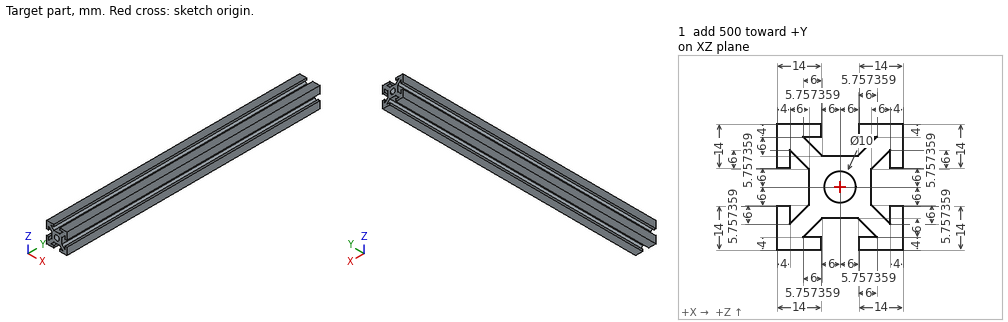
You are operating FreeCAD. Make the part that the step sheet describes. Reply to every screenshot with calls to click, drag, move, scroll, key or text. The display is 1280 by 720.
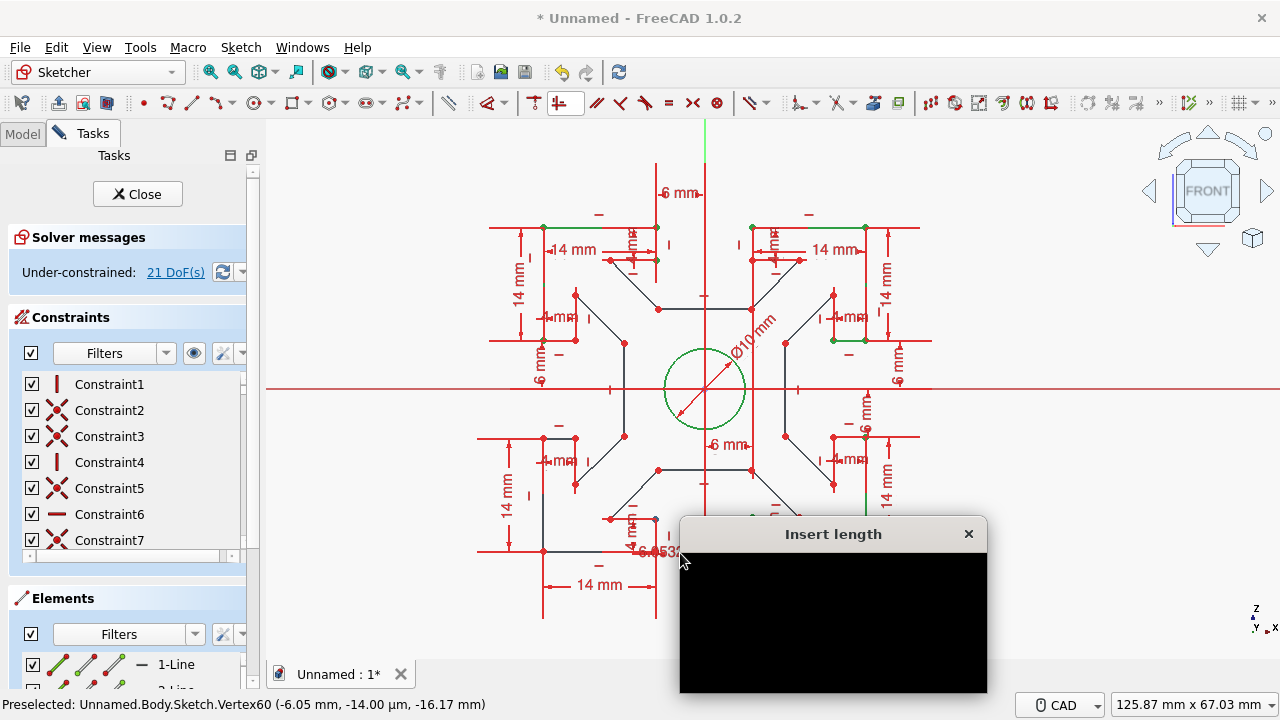
text(6)
key(Return)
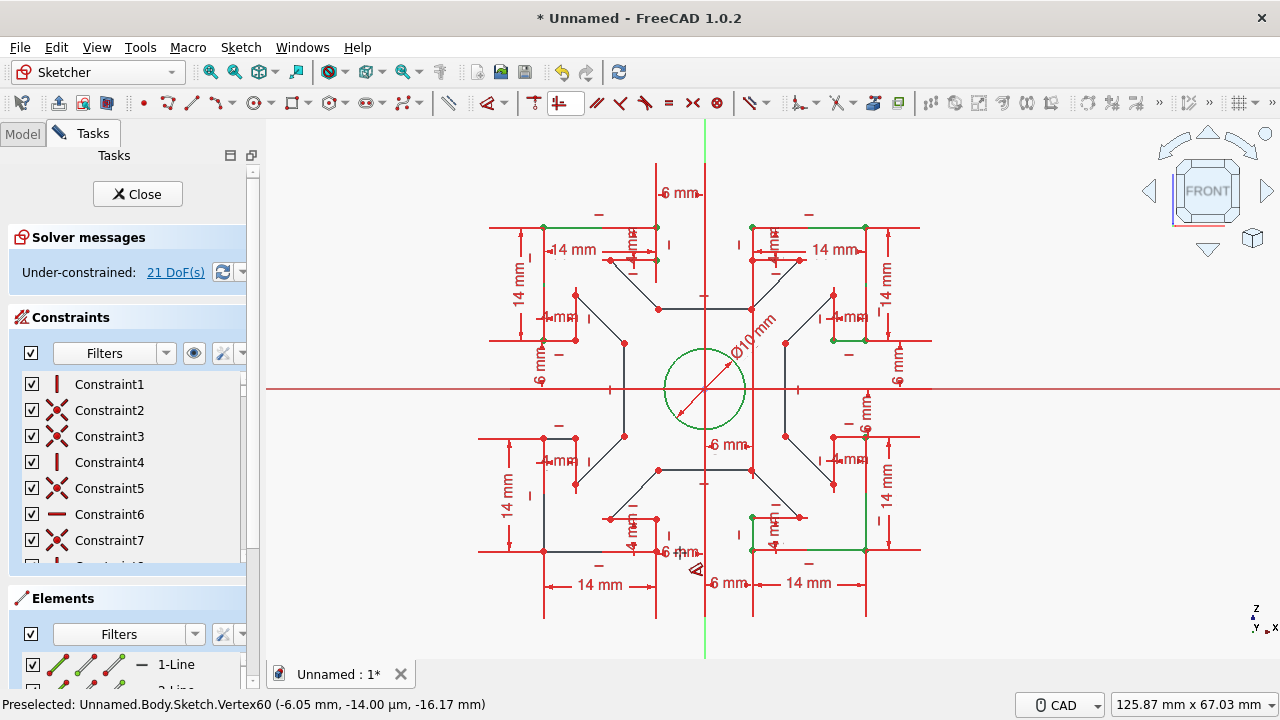
click(544, 439)
click(510, 414)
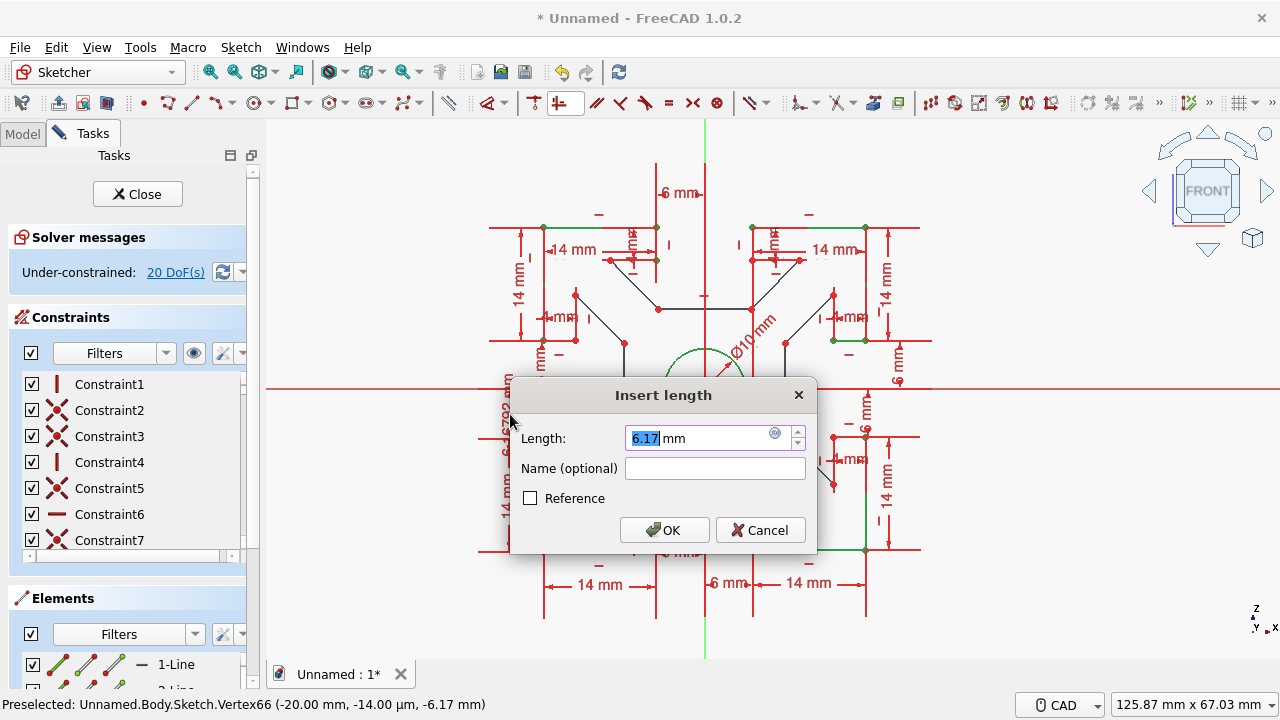
text(6)
key(Return)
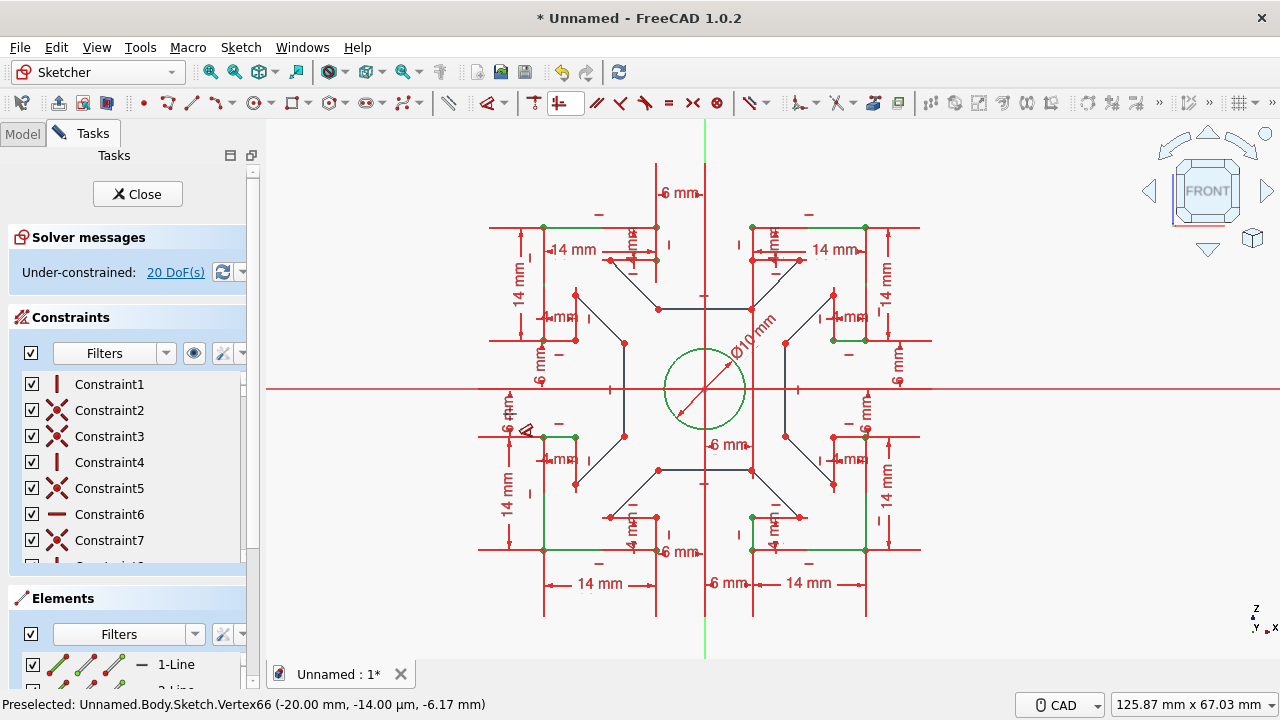
click(610, 329)
click(600, 213)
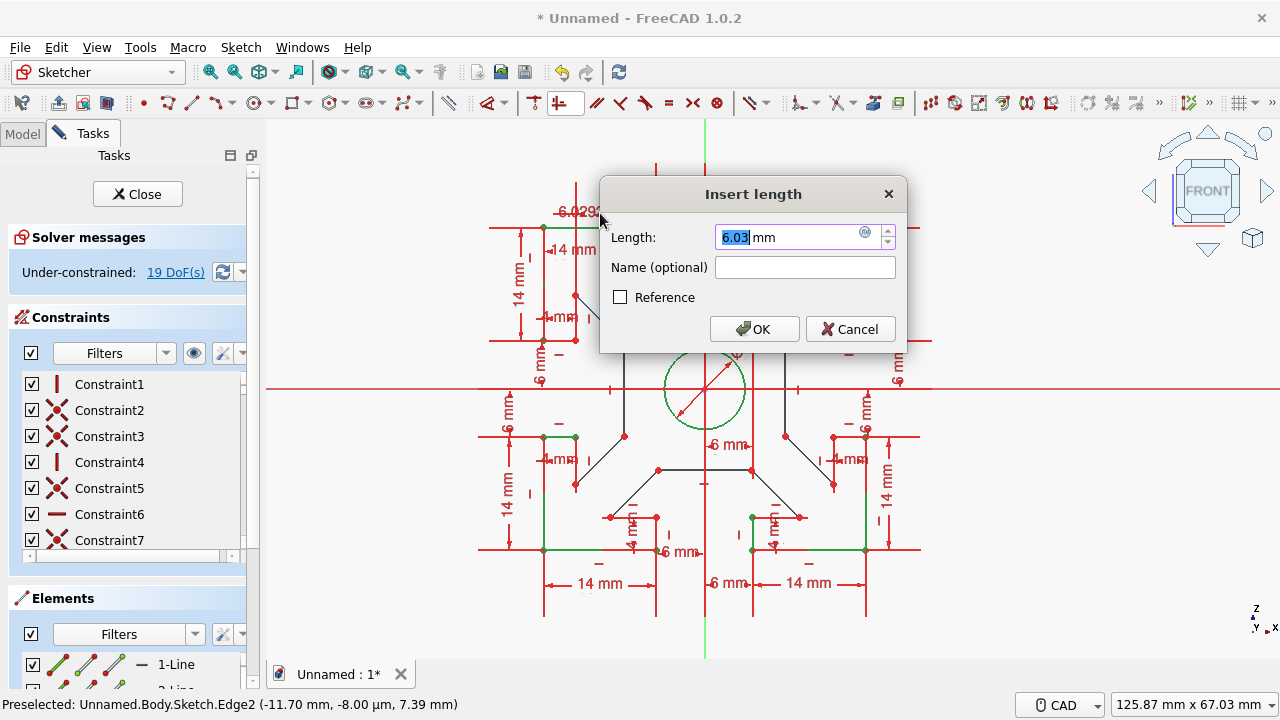
text(6)
key(Return)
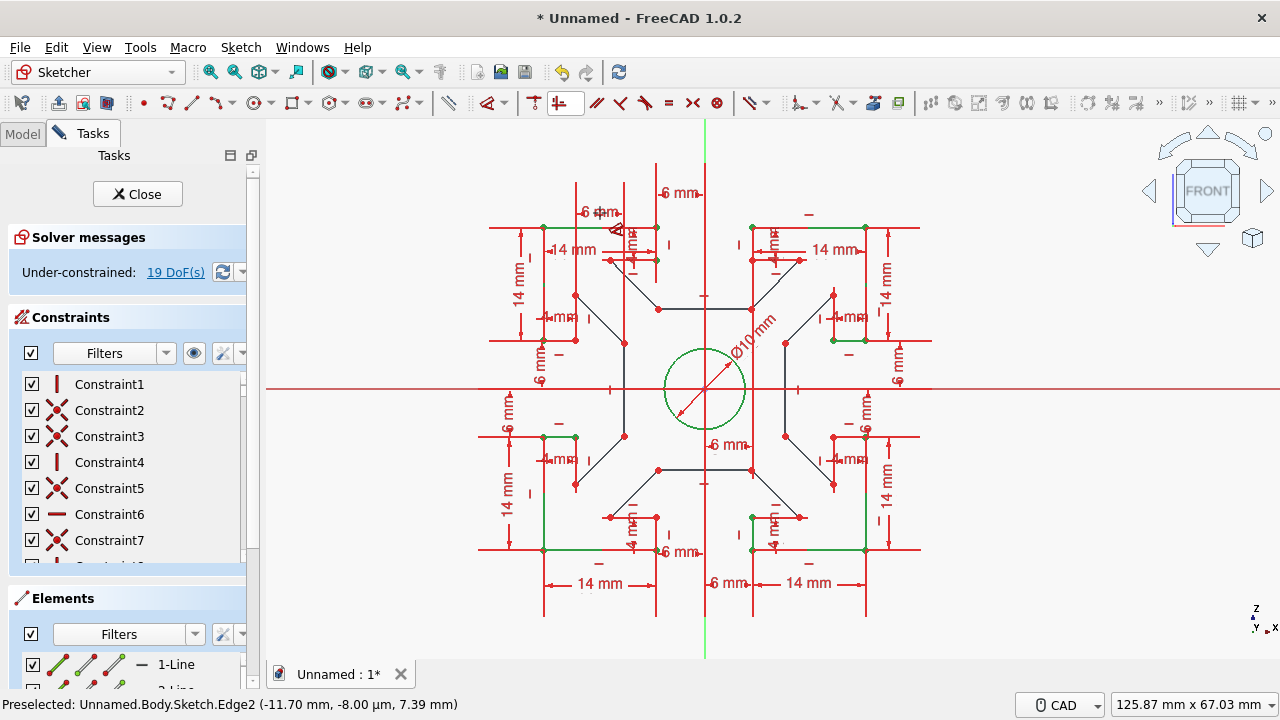
click(610, 329)
click(658, 330)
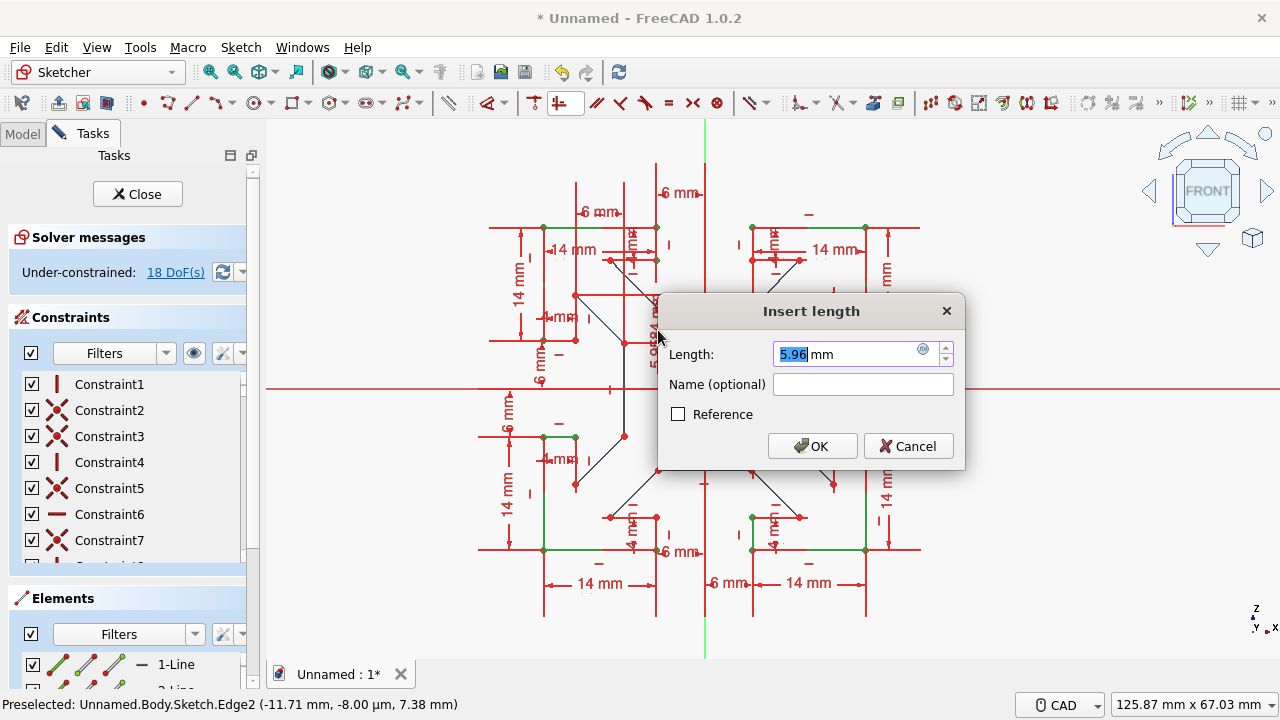
text(6)
key(Return)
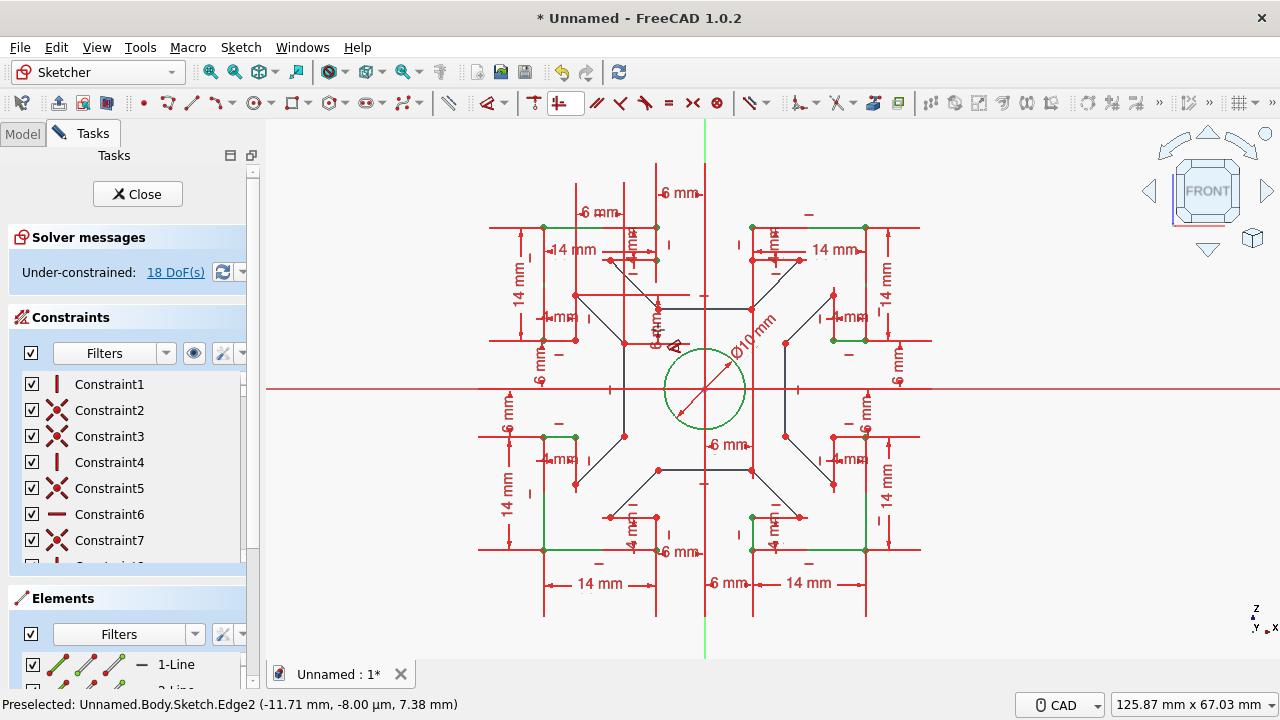
click(625, 275)
click(645, 367)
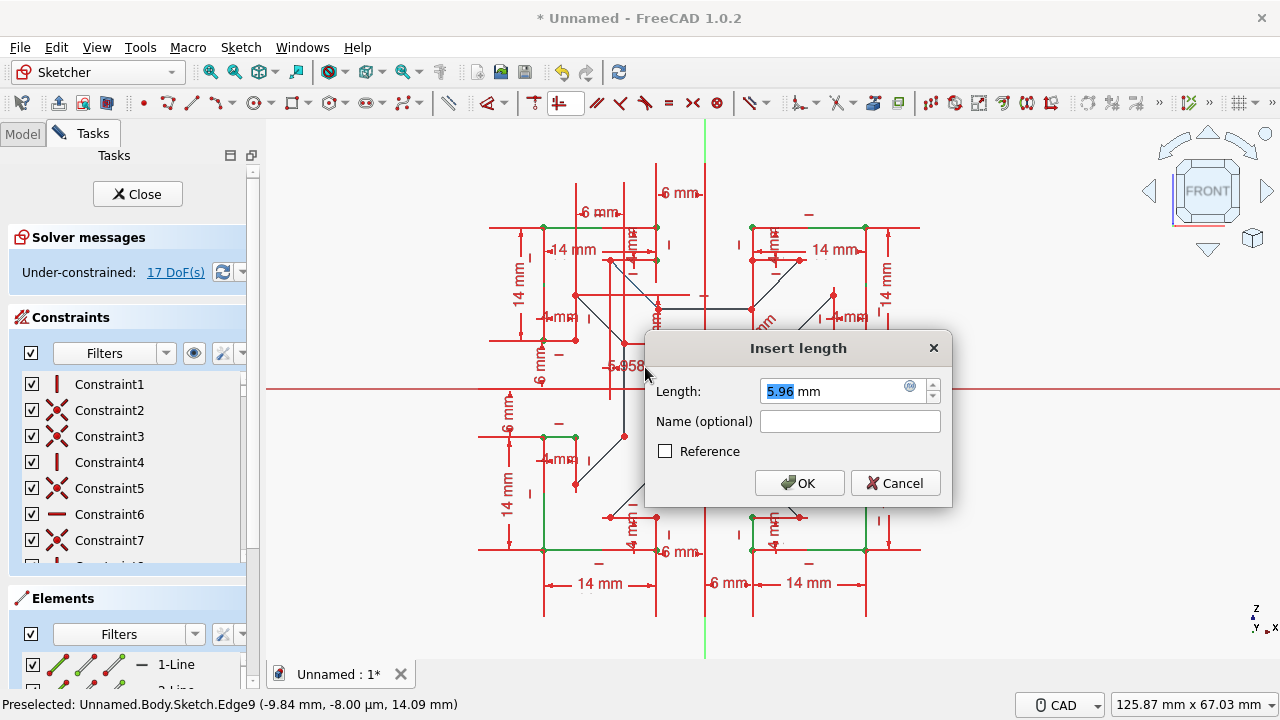
text(6)
key(Return)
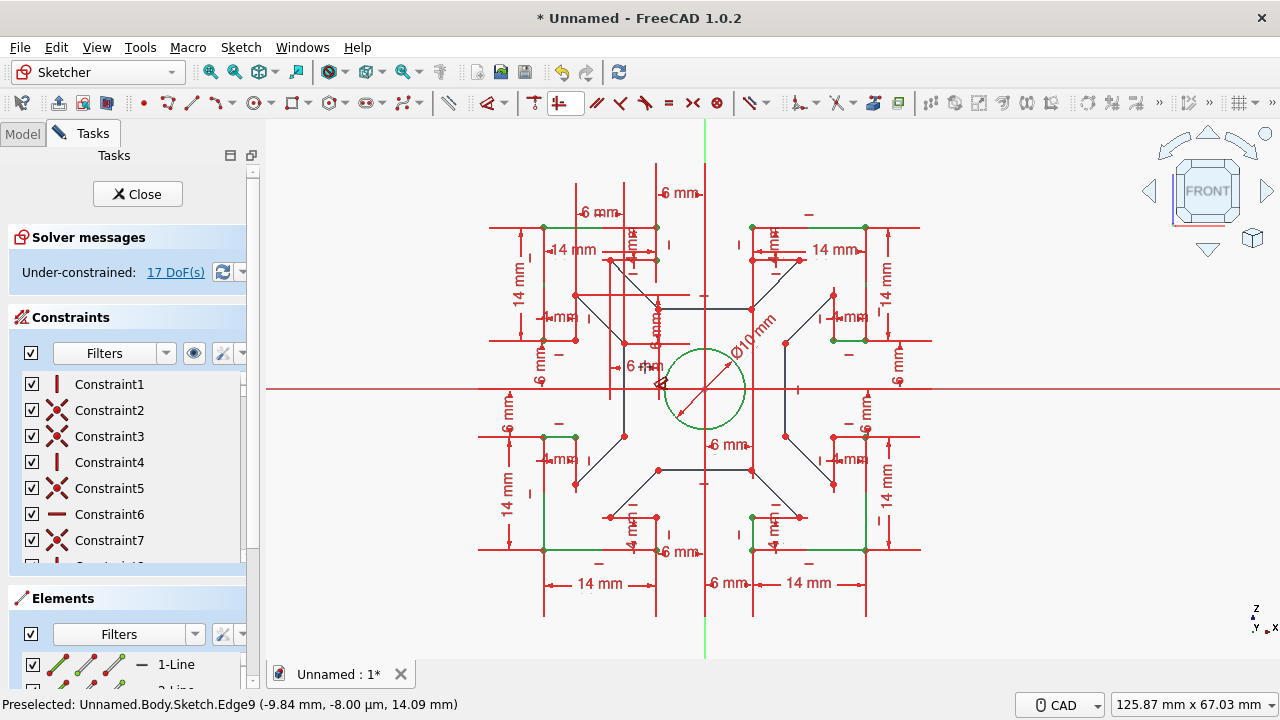
click(625, 275)
click(741, 285)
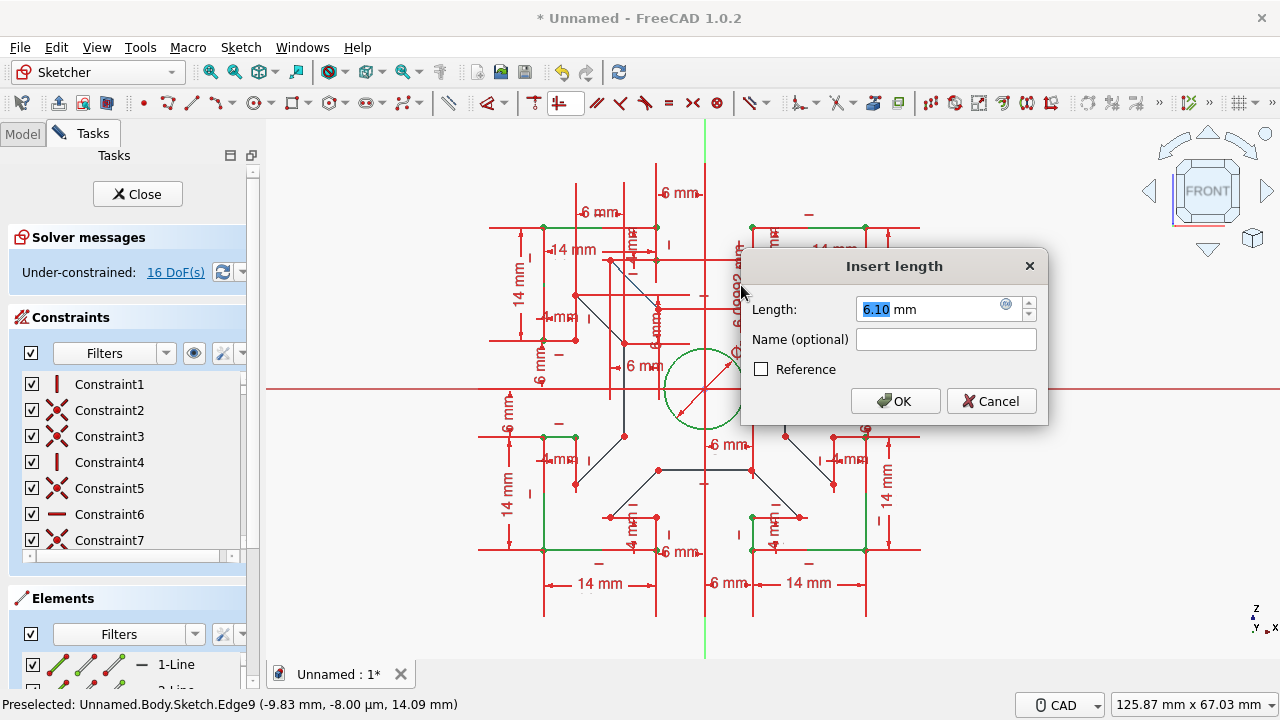
text(6)
key(Return)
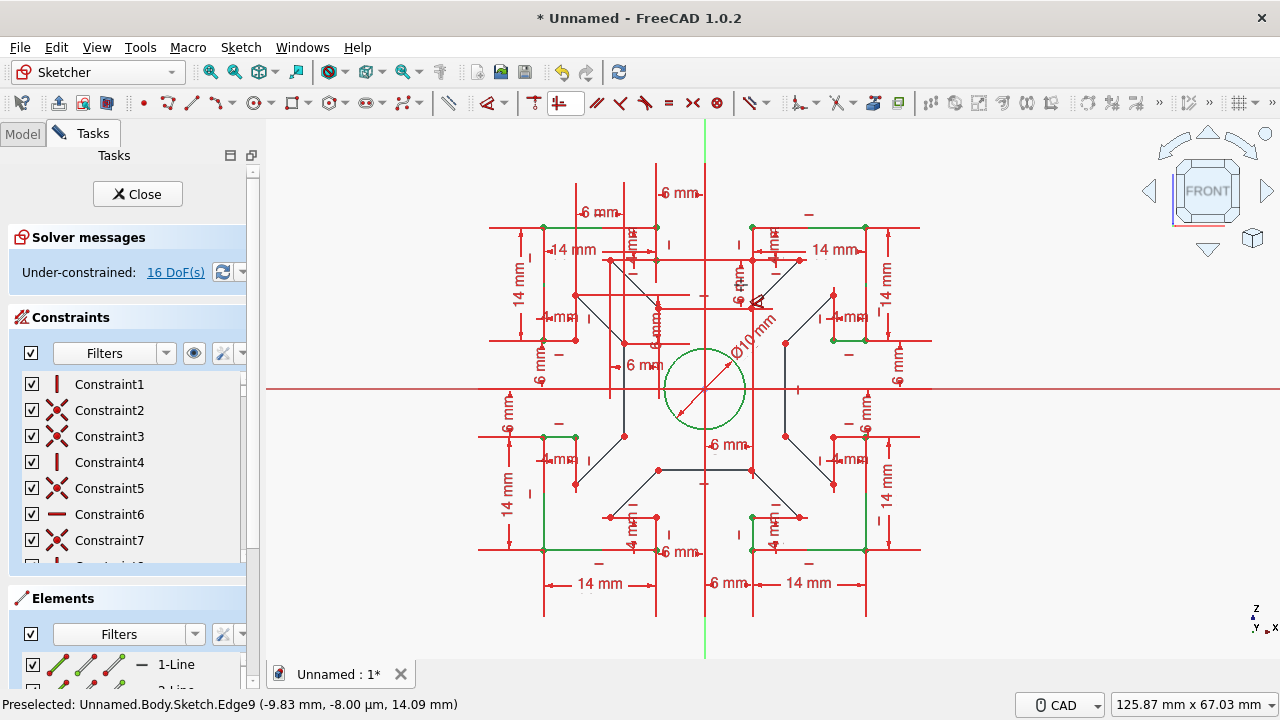
click(766, 294)
click(775, 202)